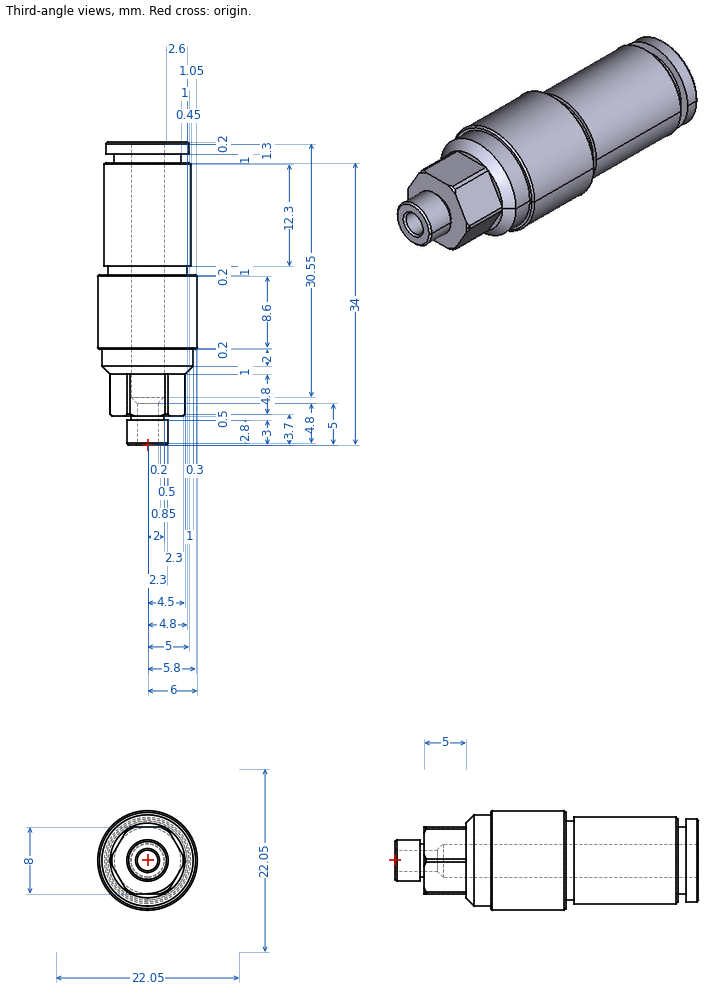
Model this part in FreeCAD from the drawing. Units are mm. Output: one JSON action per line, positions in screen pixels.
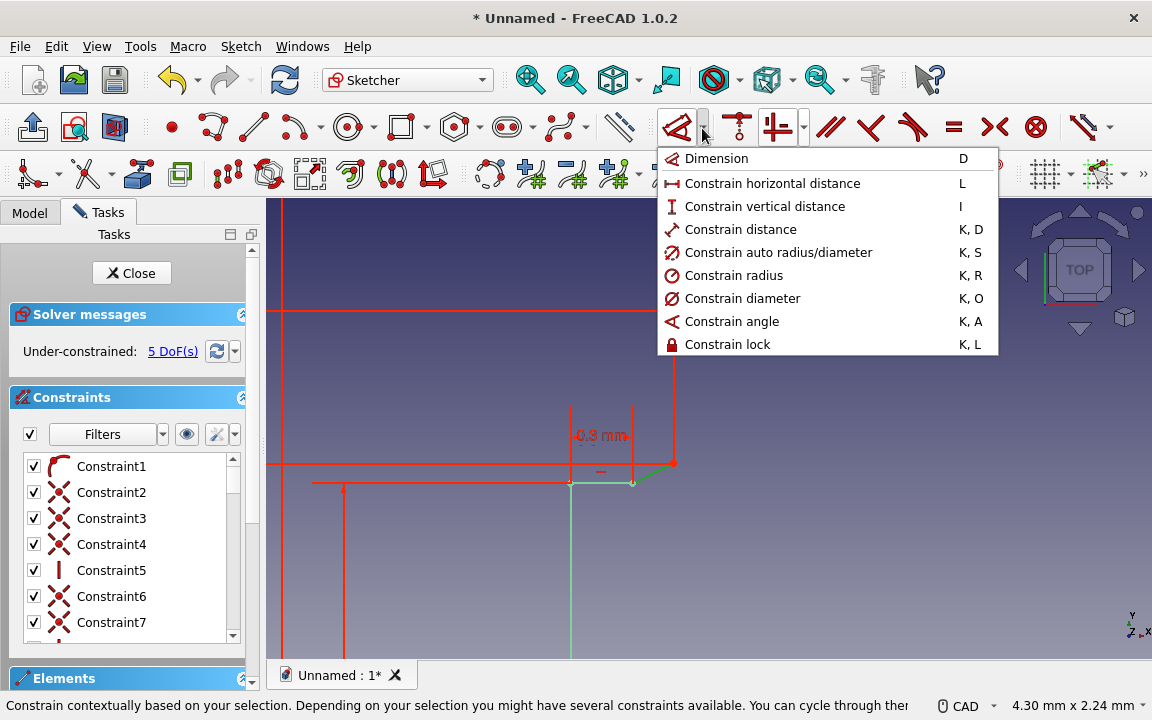
{"action": "left_click", "coordinate": [828, 206]}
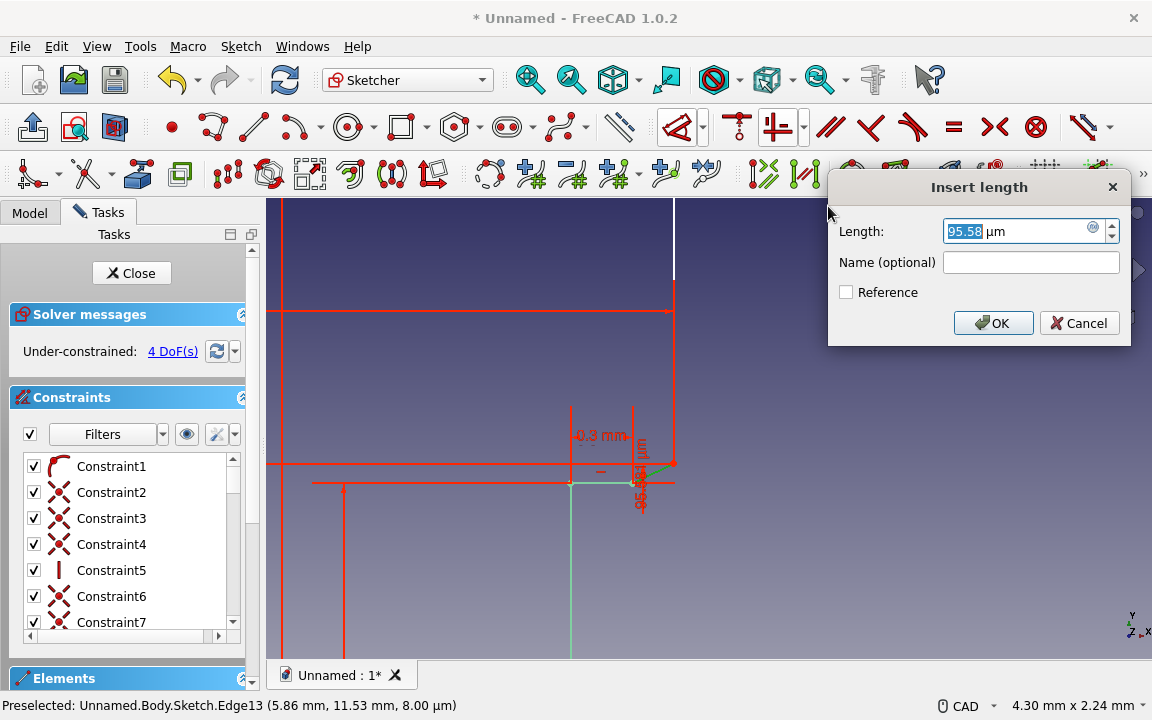
{"action": "key", "text": "ctrl+a"}
{"action": "type", "text": "0.2 mm"}
{"action": "key", "text": "Return"}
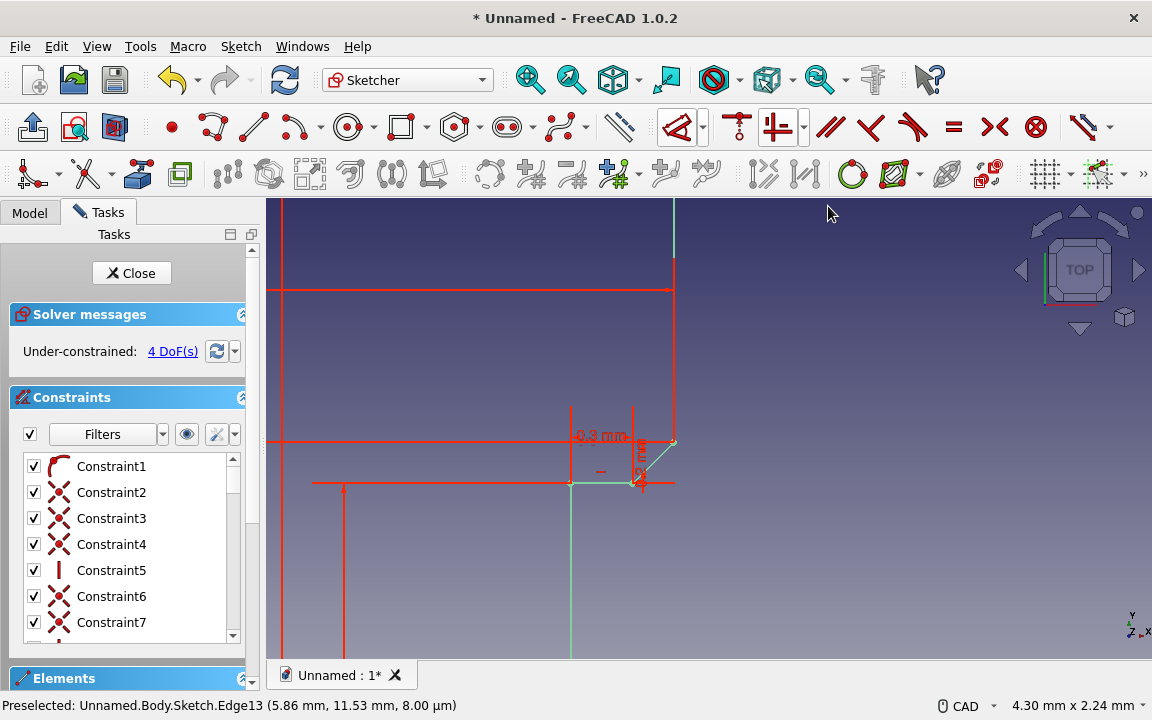
{"action": "scroll", "coordinate": [665, 485], "scroll_direction": "down", "scroll_amount": 16}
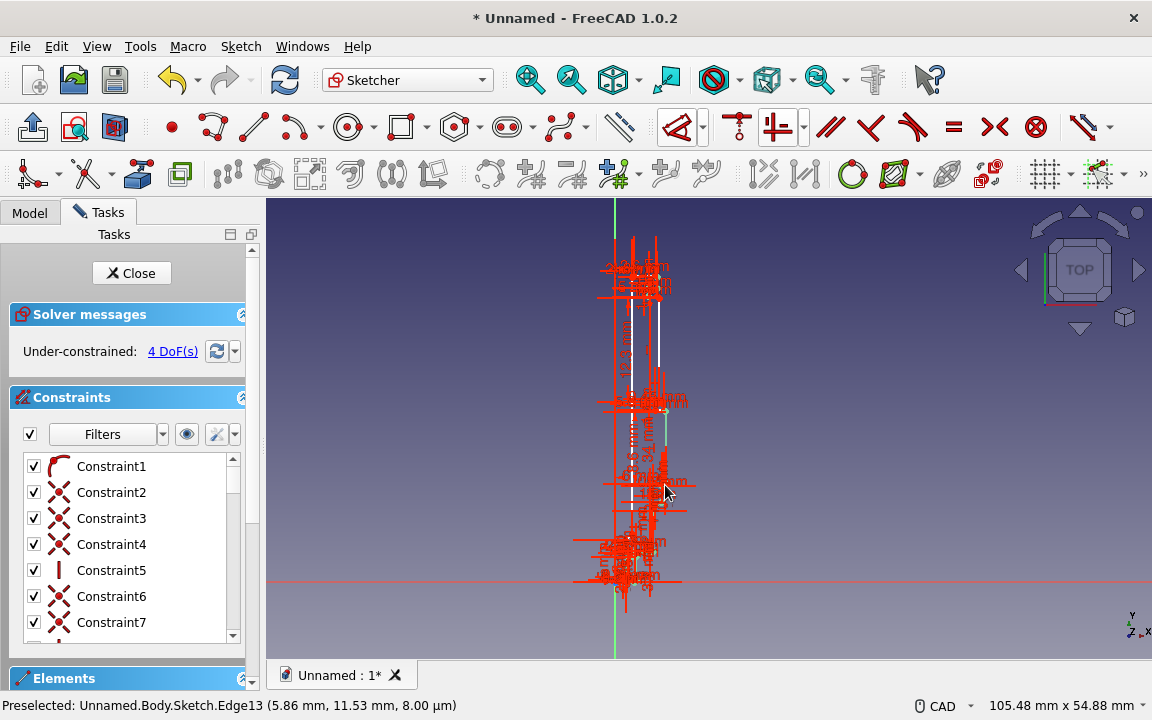
{"action": "scroll", "coordinate": [665, 411], "scroll_direction": "up", "scroll_amount": 16}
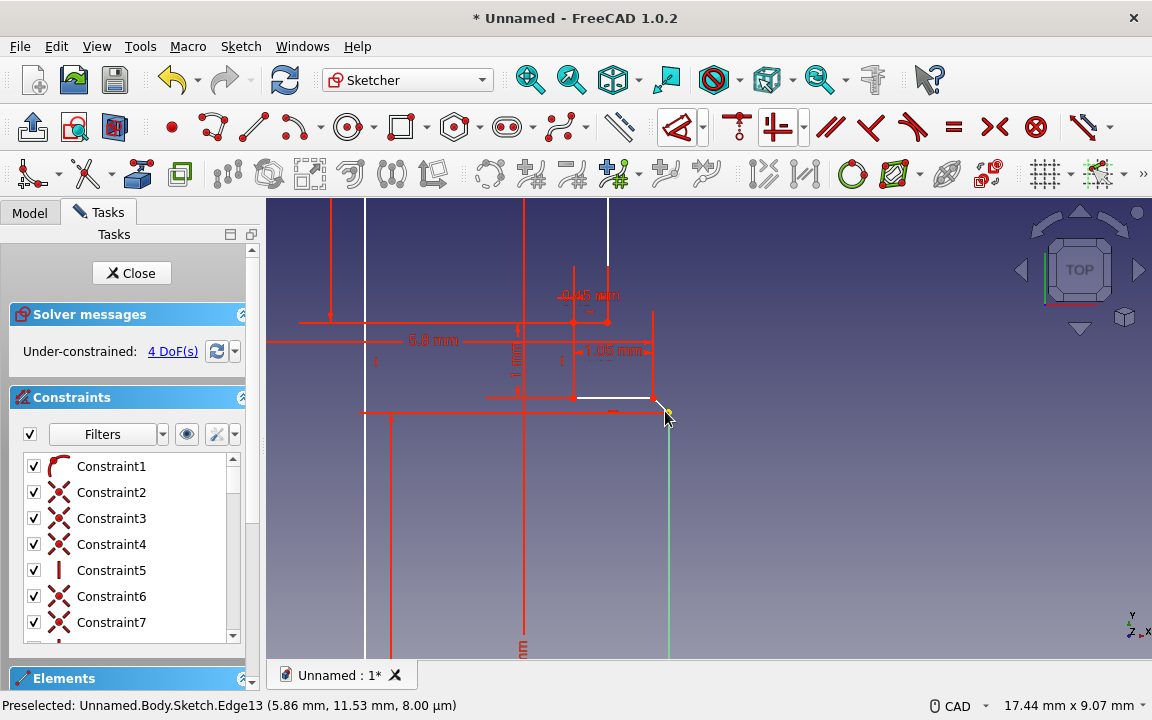
{"action": "left_click", "coordinate": [661, 403]}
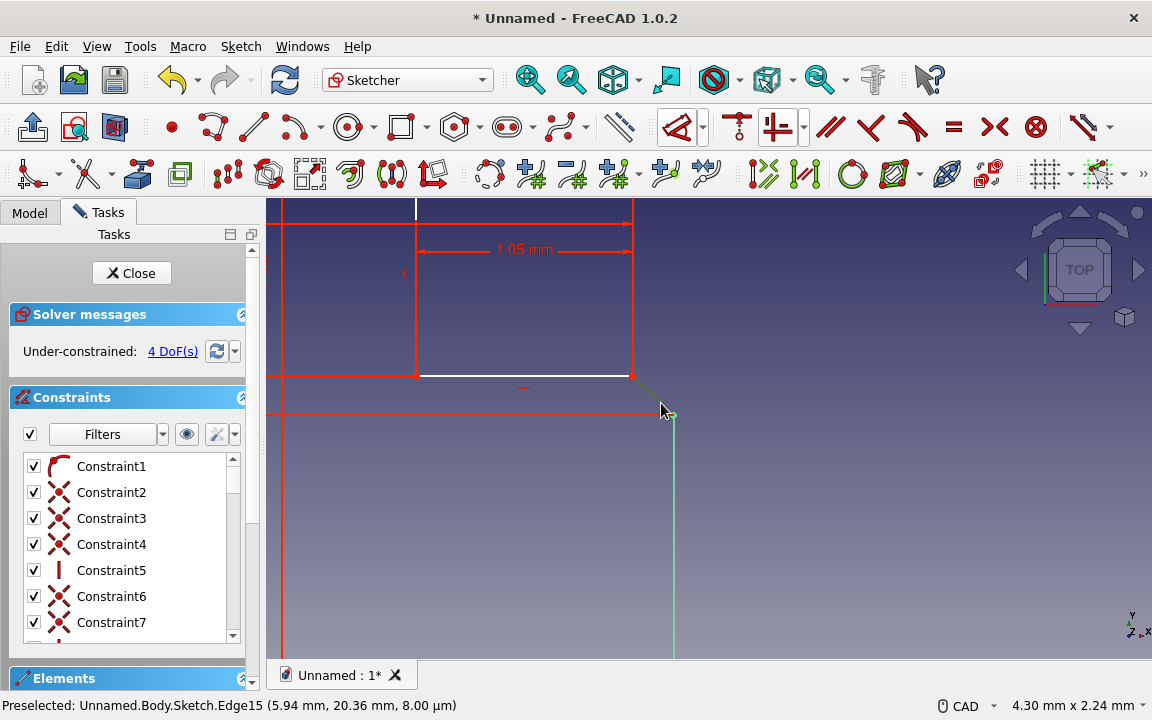
{"action": "key", "text": "i"}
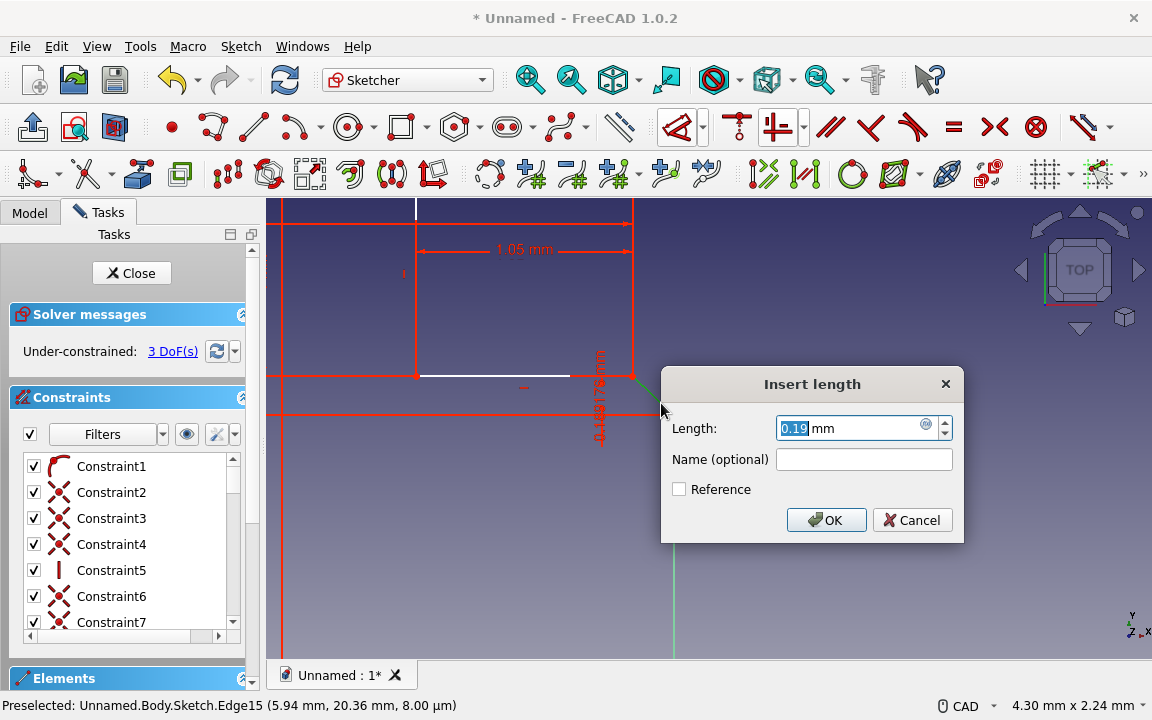
{"action": "type", "text": "0.2"}
{"action": "key", "text": "Return"}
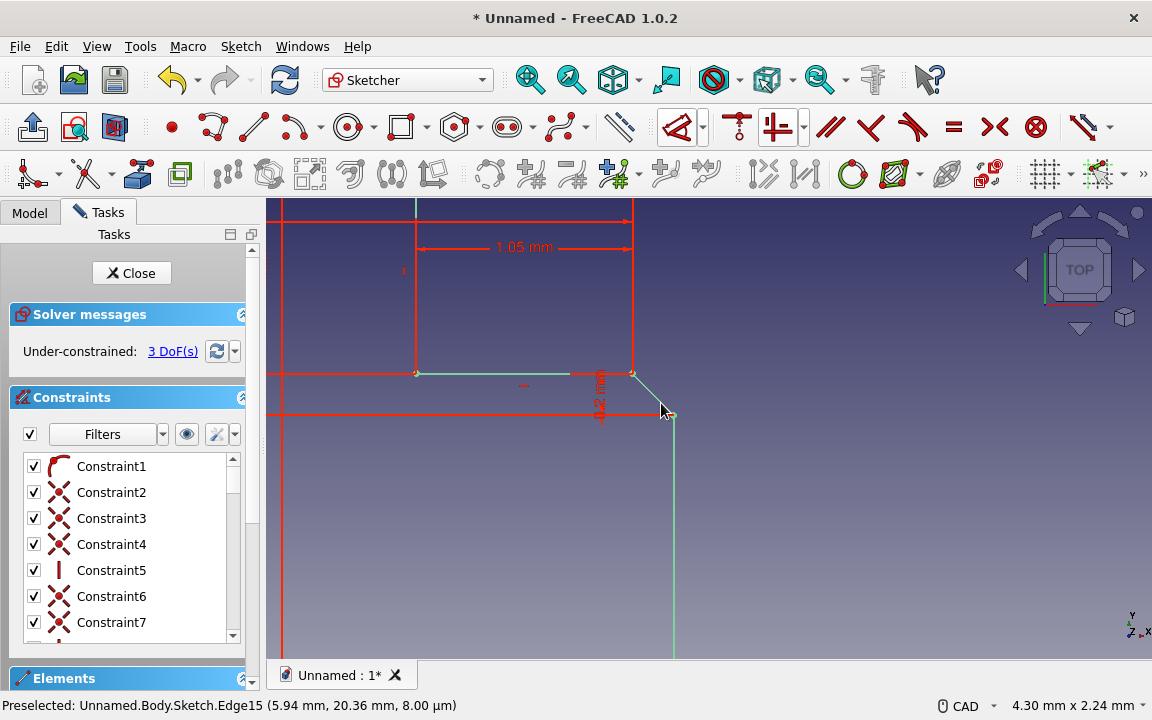
{"action": "scroll", "coordinate": [665, 411], "scroll_direction": "down", "scroll_amount": 16}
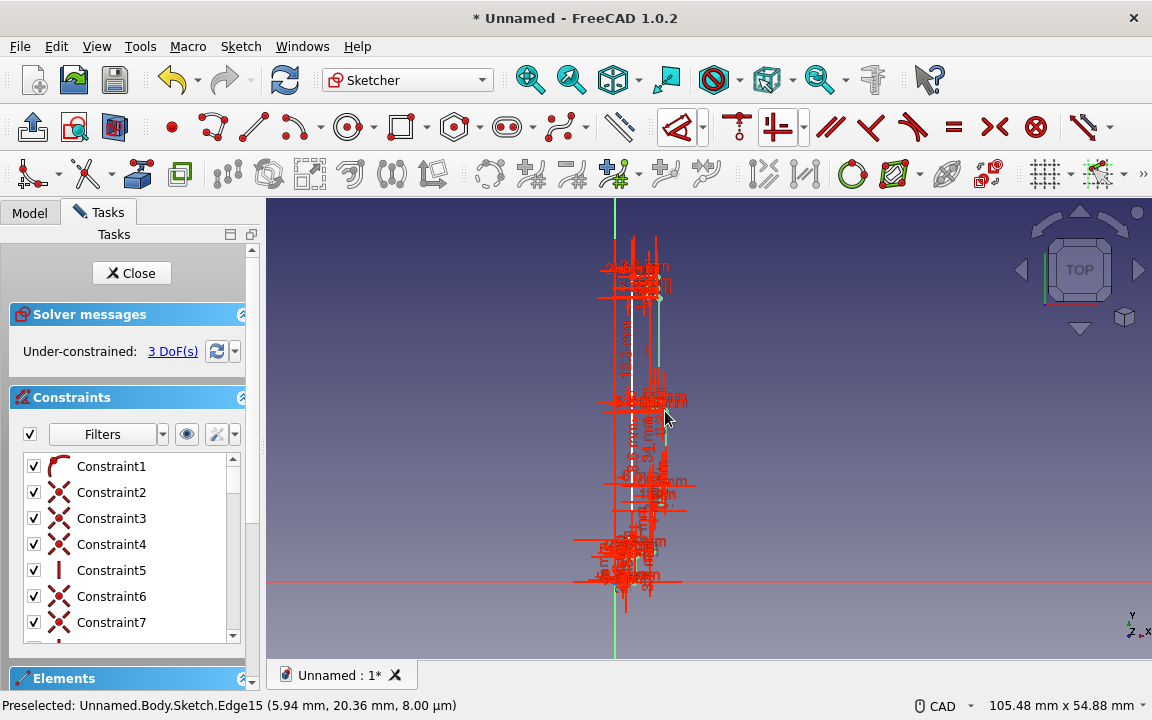
{"action": "scroll", "coordinate": [657, 277], "scroll_direction": "up", "scroll_amount": 16}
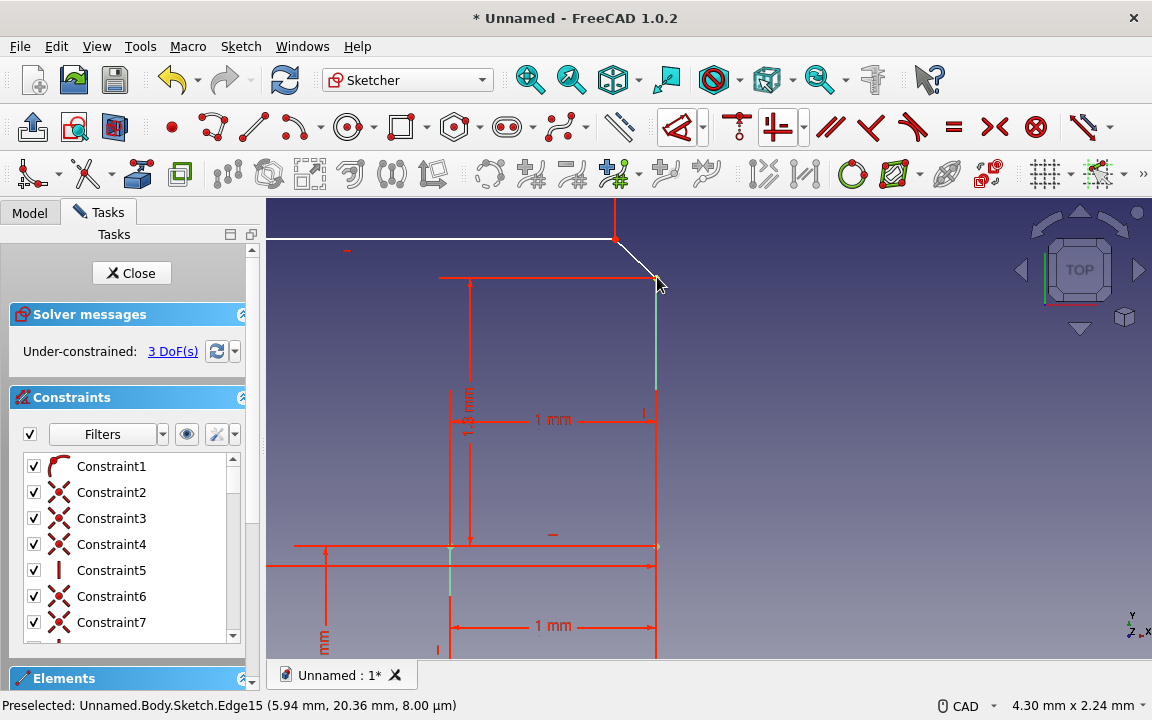
{"action": "left_click", "coordinate": [644, 267]}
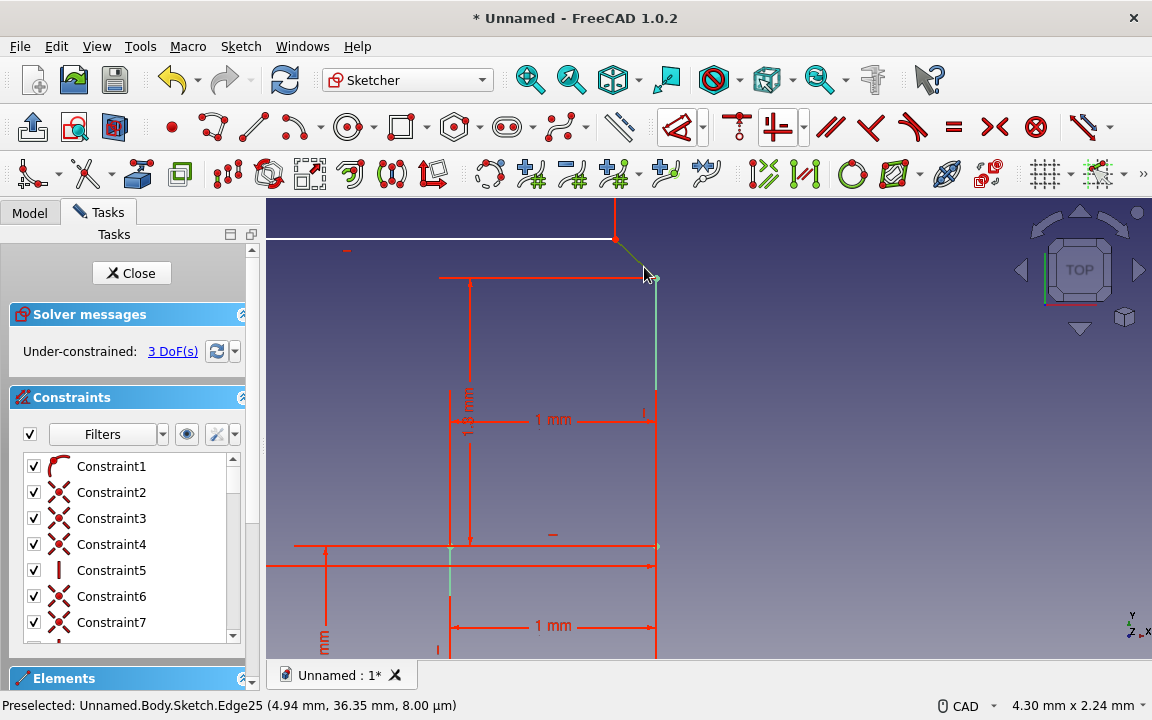
{"action": "key", "text": "i"}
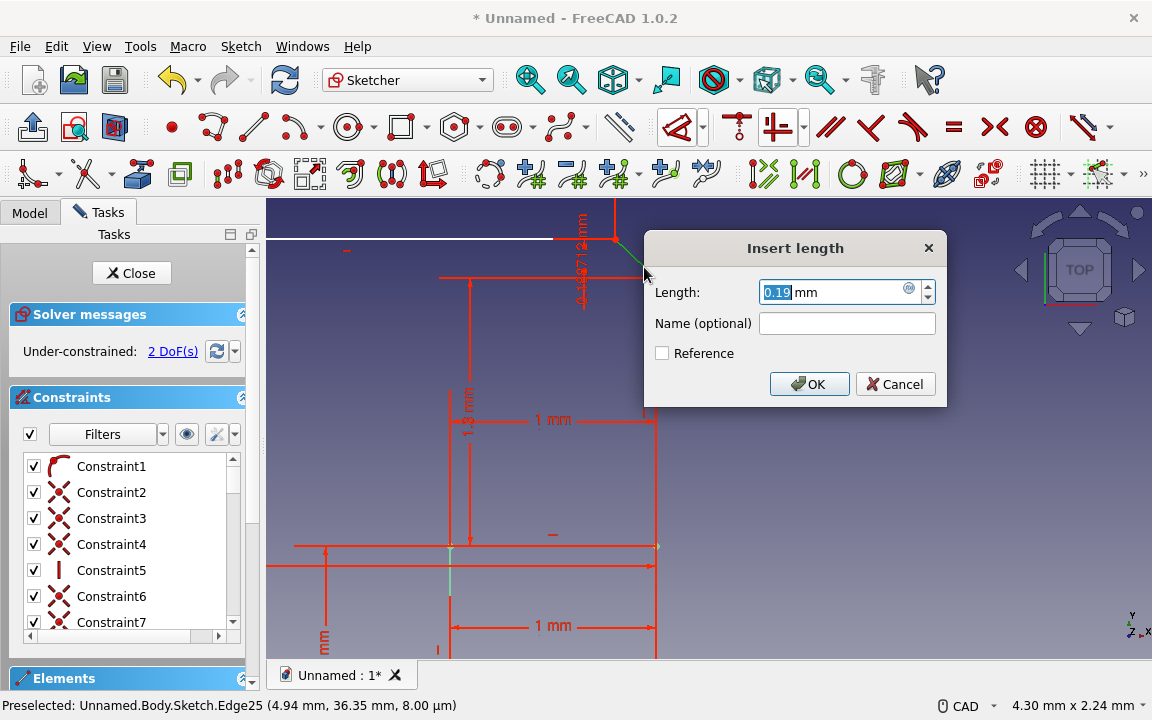
{"action": "type", "text": "0.2"}
{"action": "key", "text": "Return"}